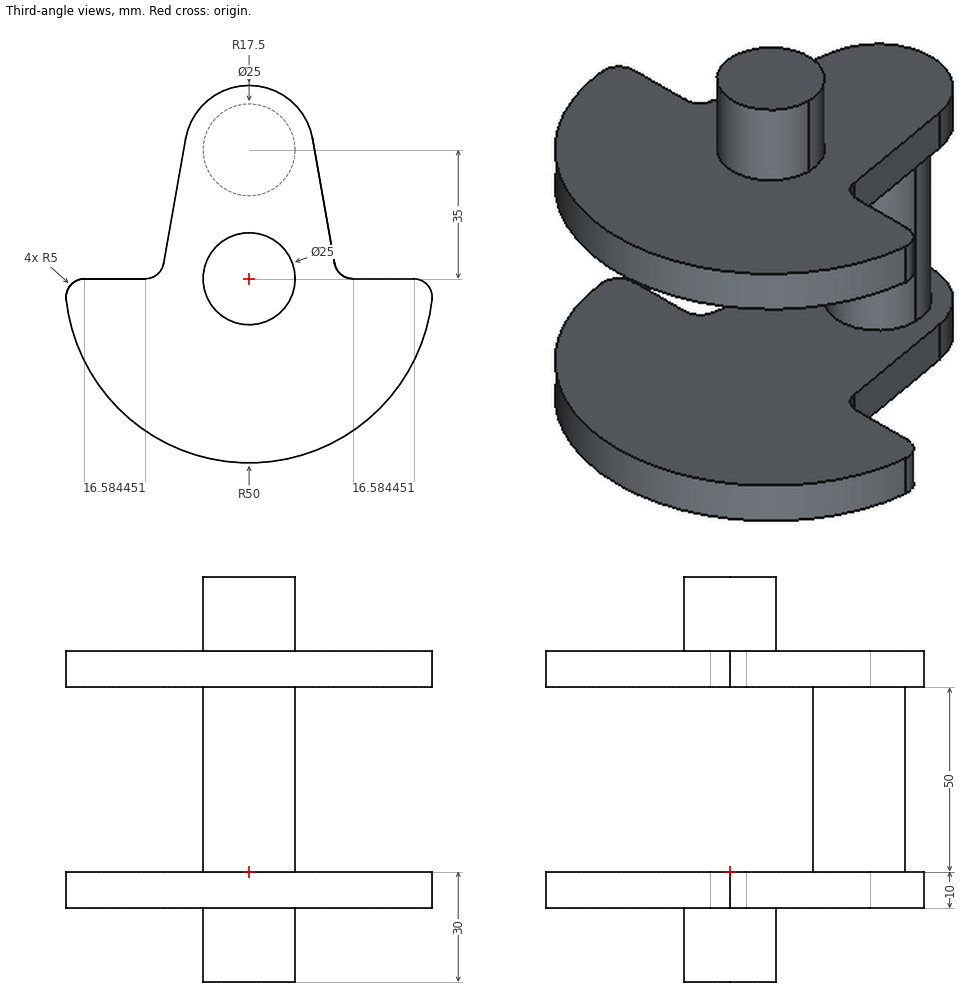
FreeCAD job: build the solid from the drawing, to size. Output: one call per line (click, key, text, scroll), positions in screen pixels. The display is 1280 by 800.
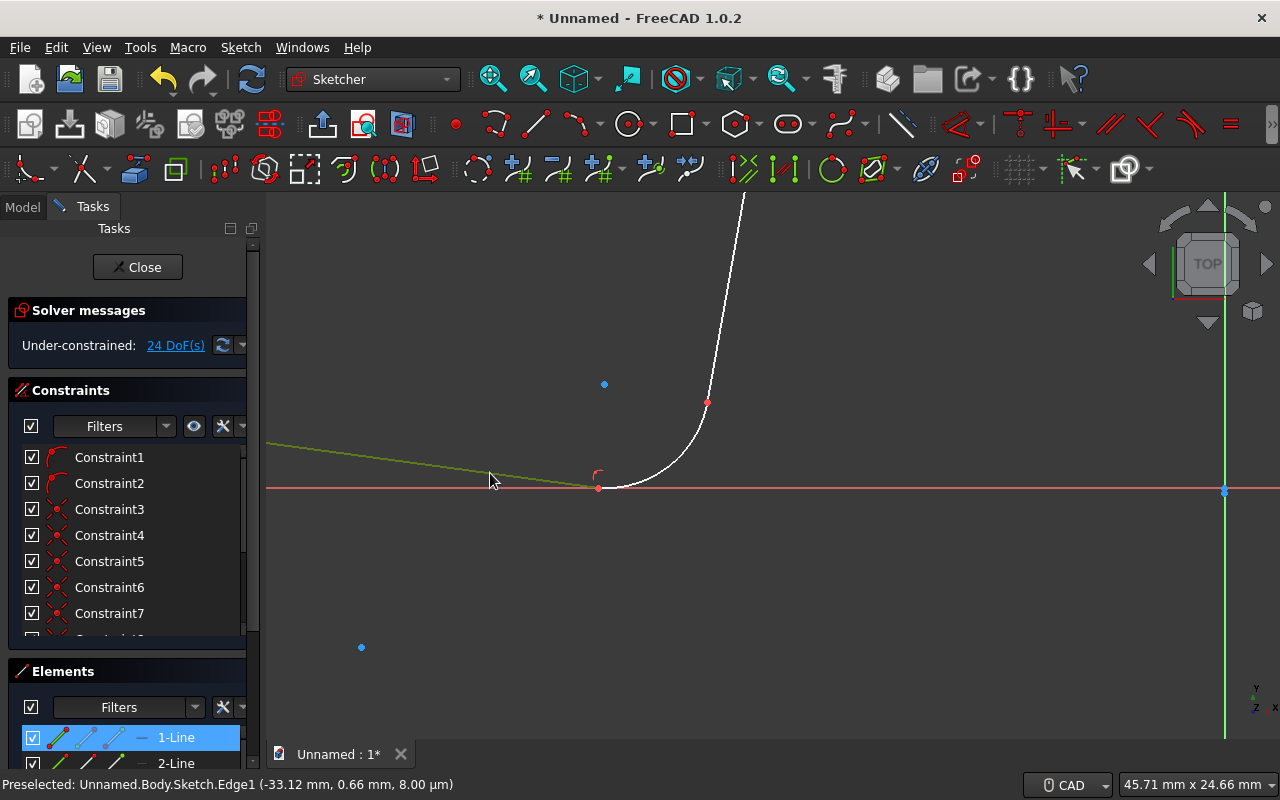
scroll(601, 467, down, 9)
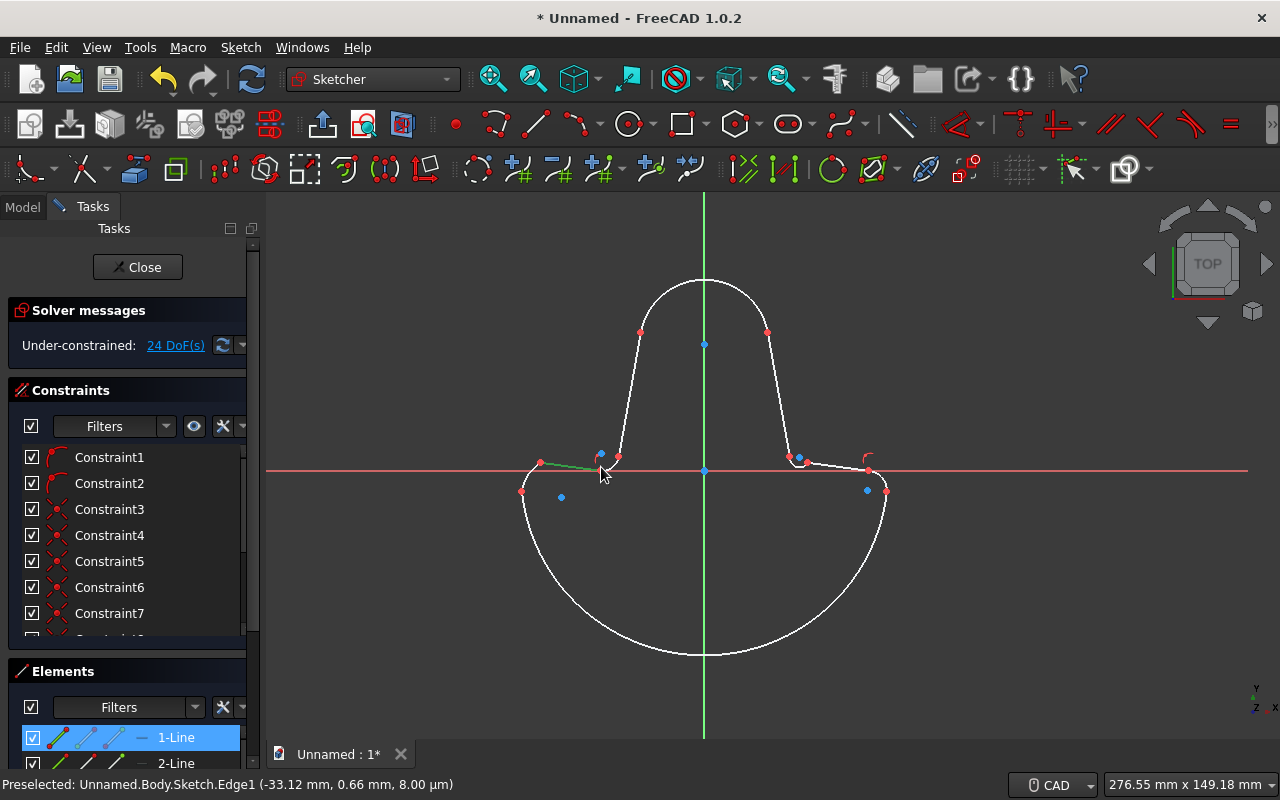
scroll(525, 481, up, 2)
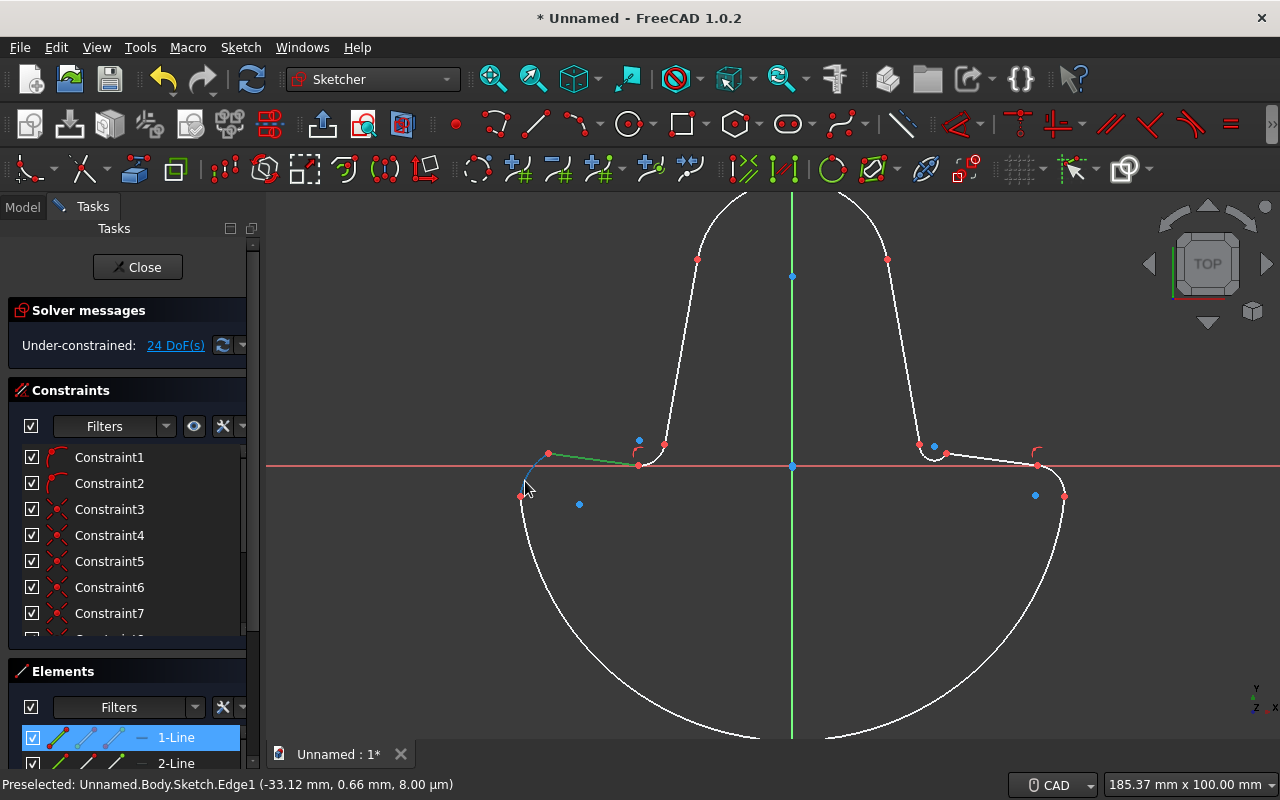
click(524, 481)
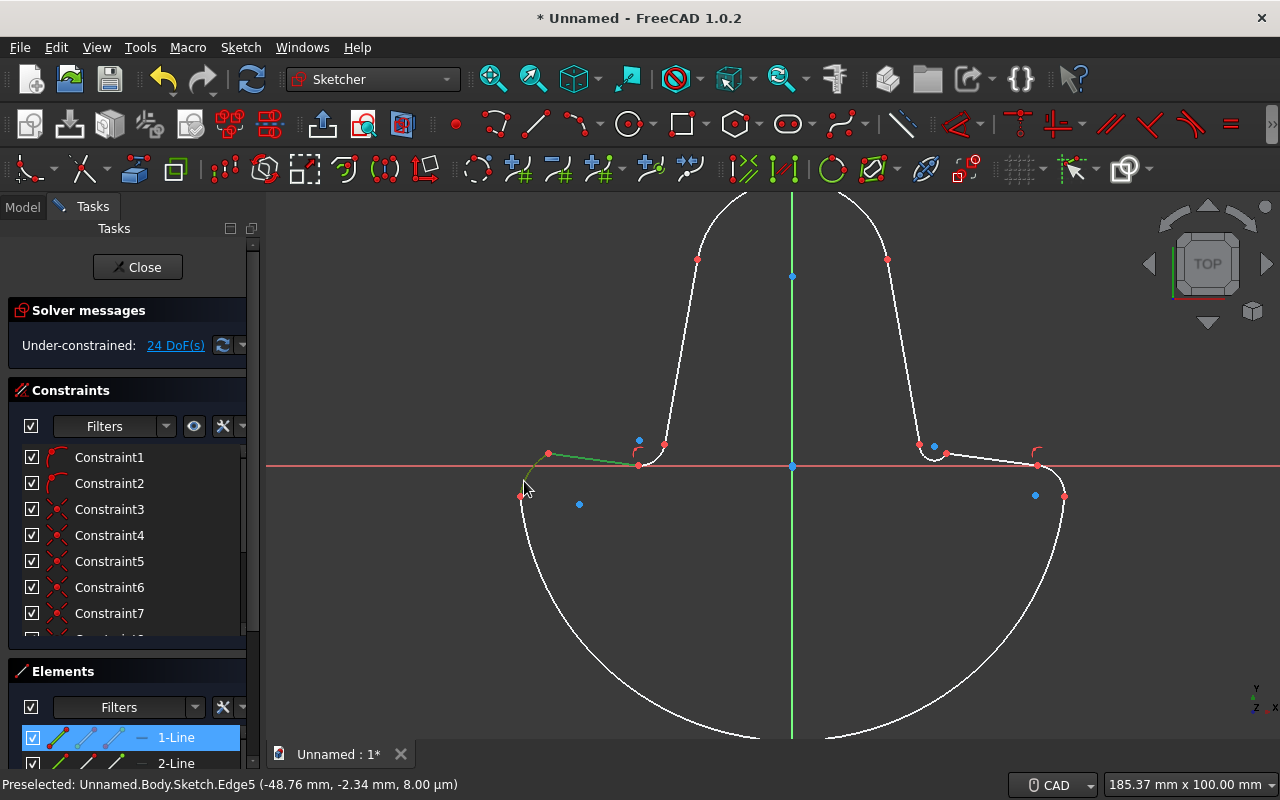
key(t)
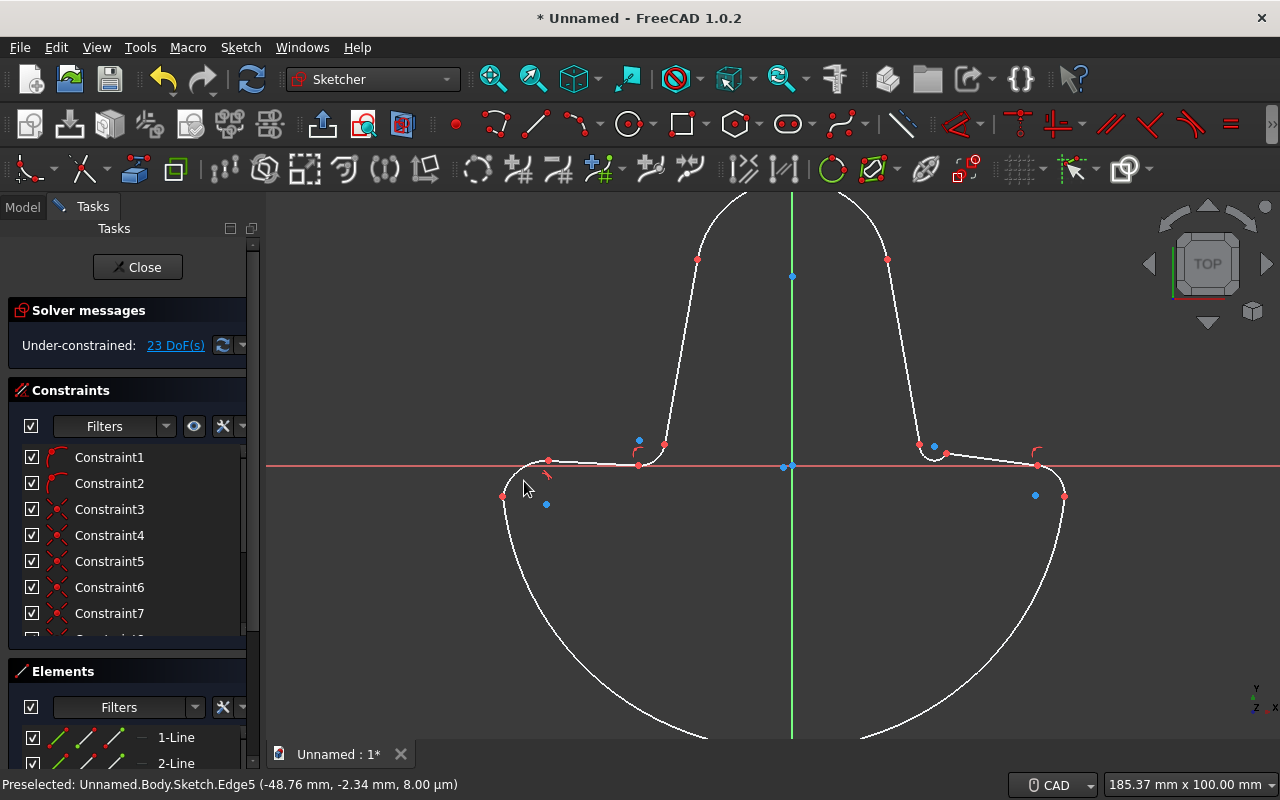
click(611, 464)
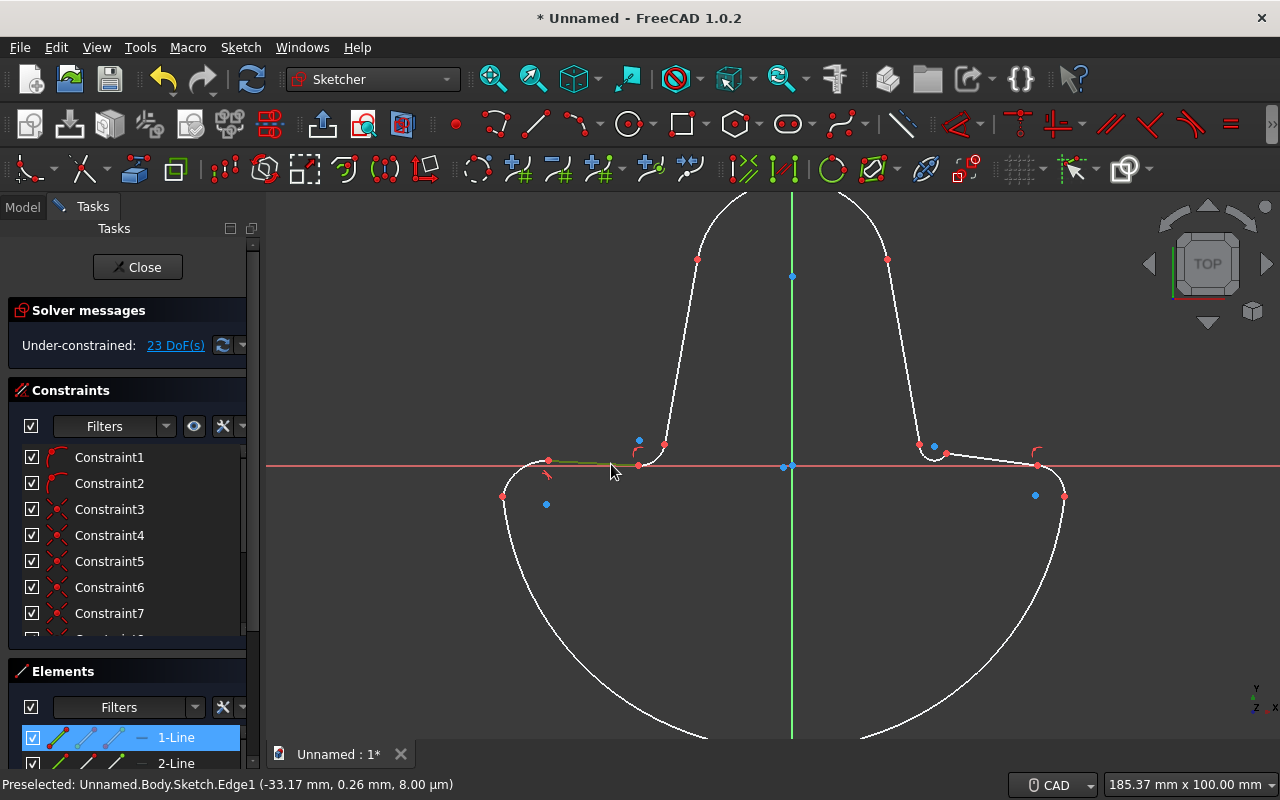
scroll(649, 464, up, 2)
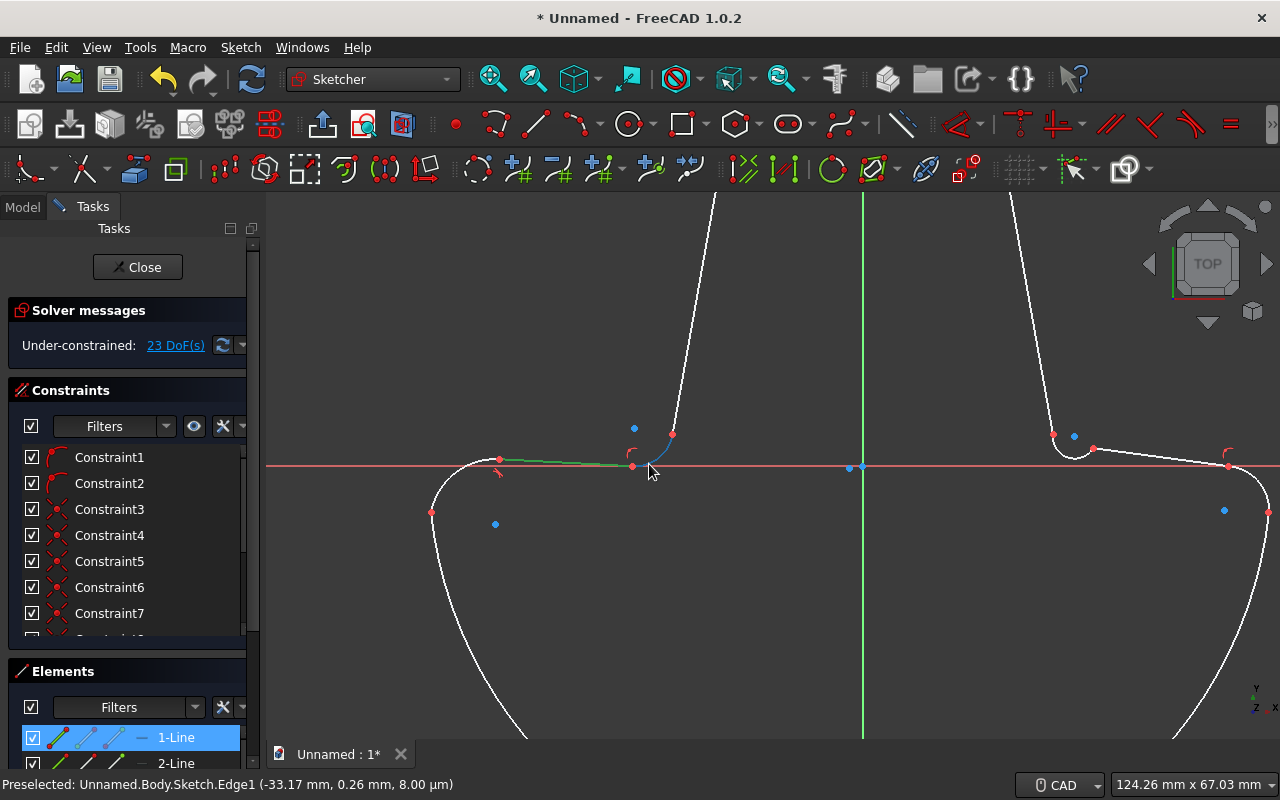
click(649, 464)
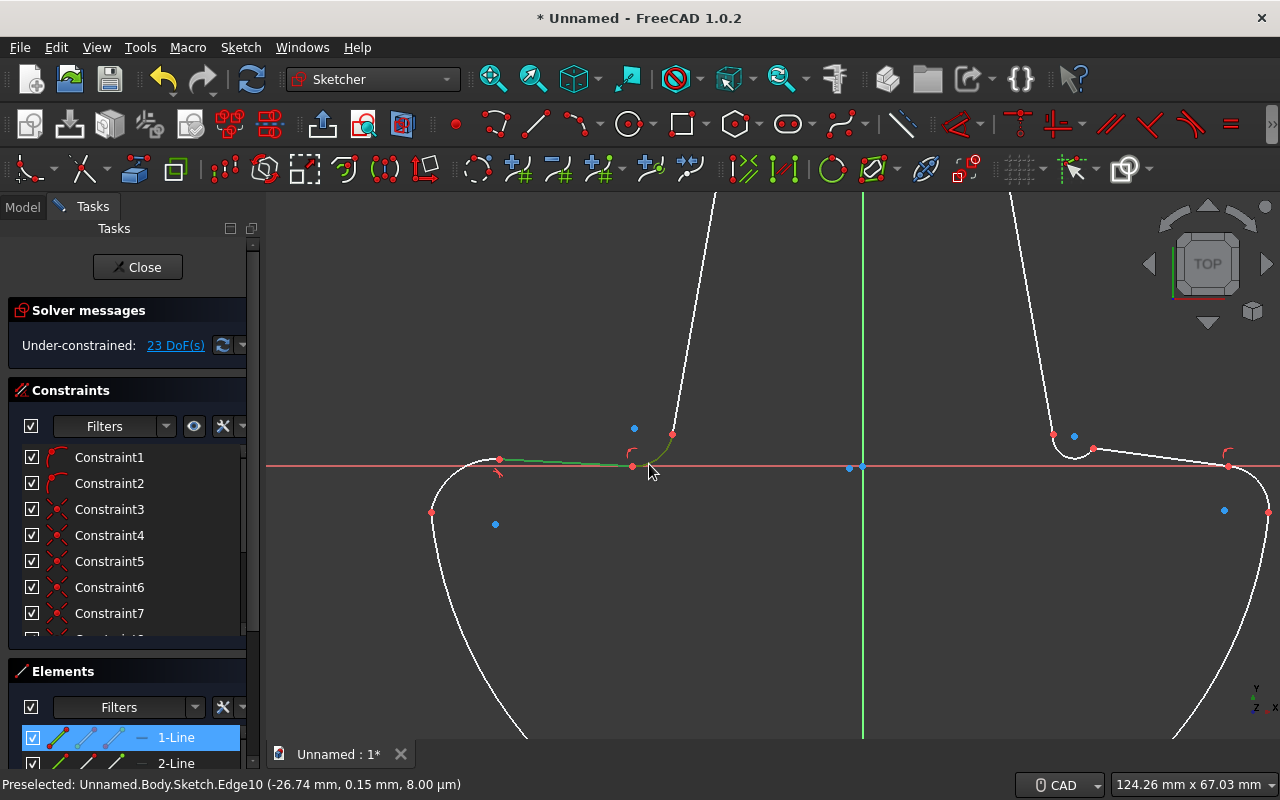
key(t)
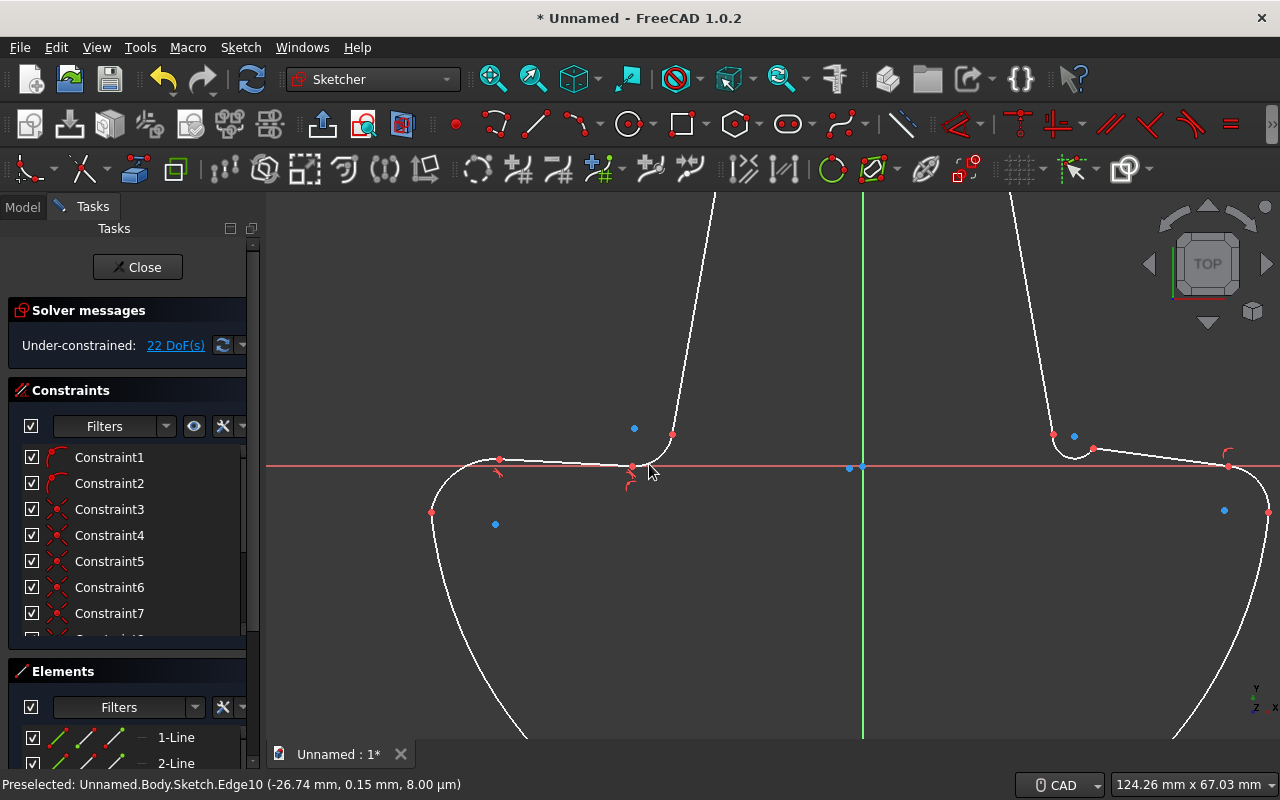
scroll(575, 473, down, 4)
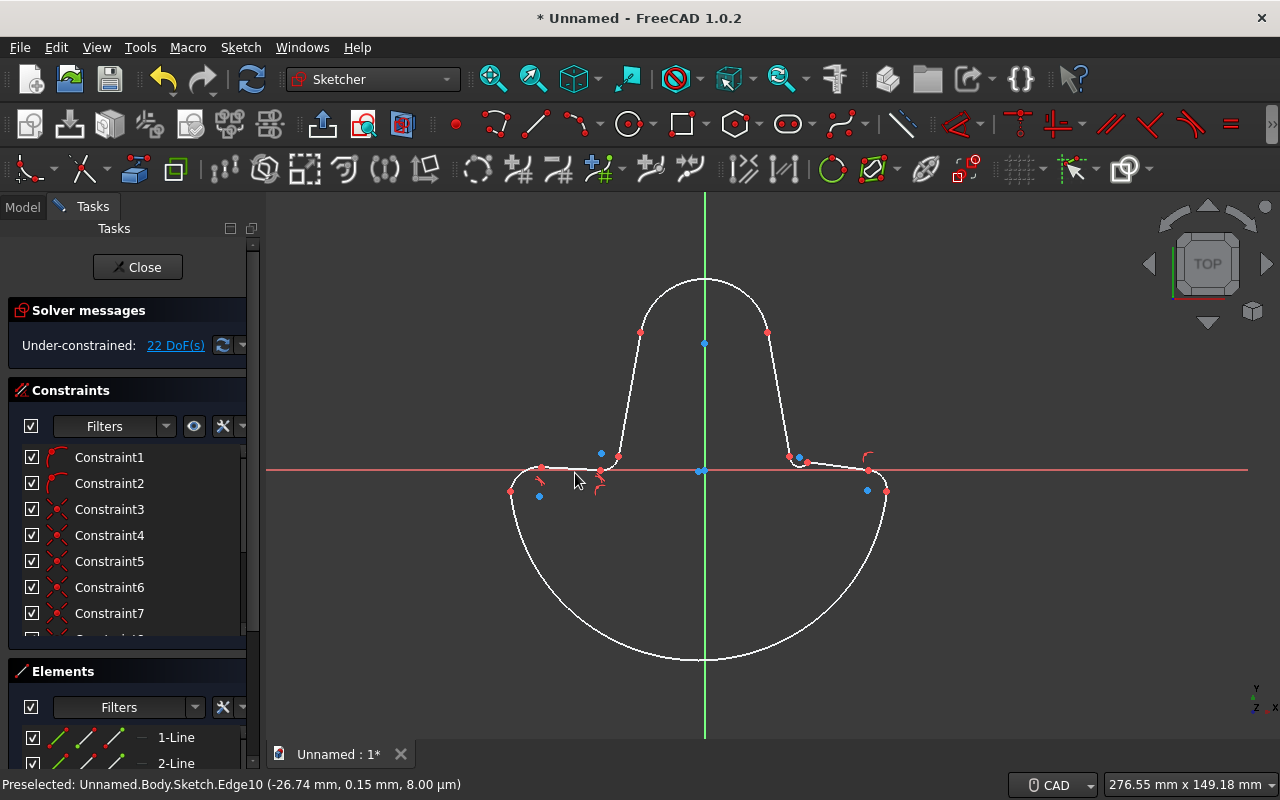
scroll(826, 465, up, 5)